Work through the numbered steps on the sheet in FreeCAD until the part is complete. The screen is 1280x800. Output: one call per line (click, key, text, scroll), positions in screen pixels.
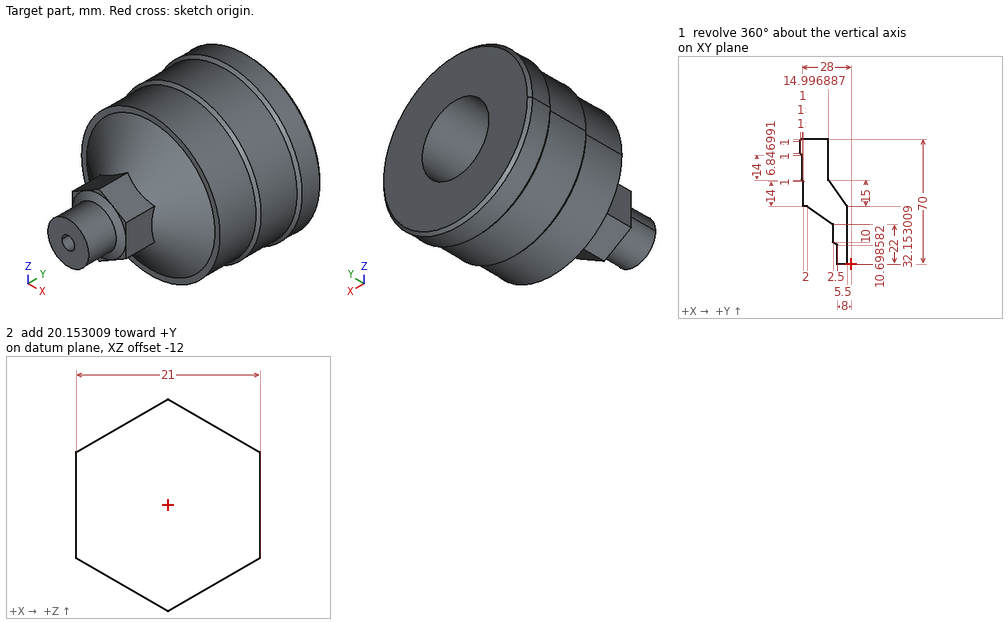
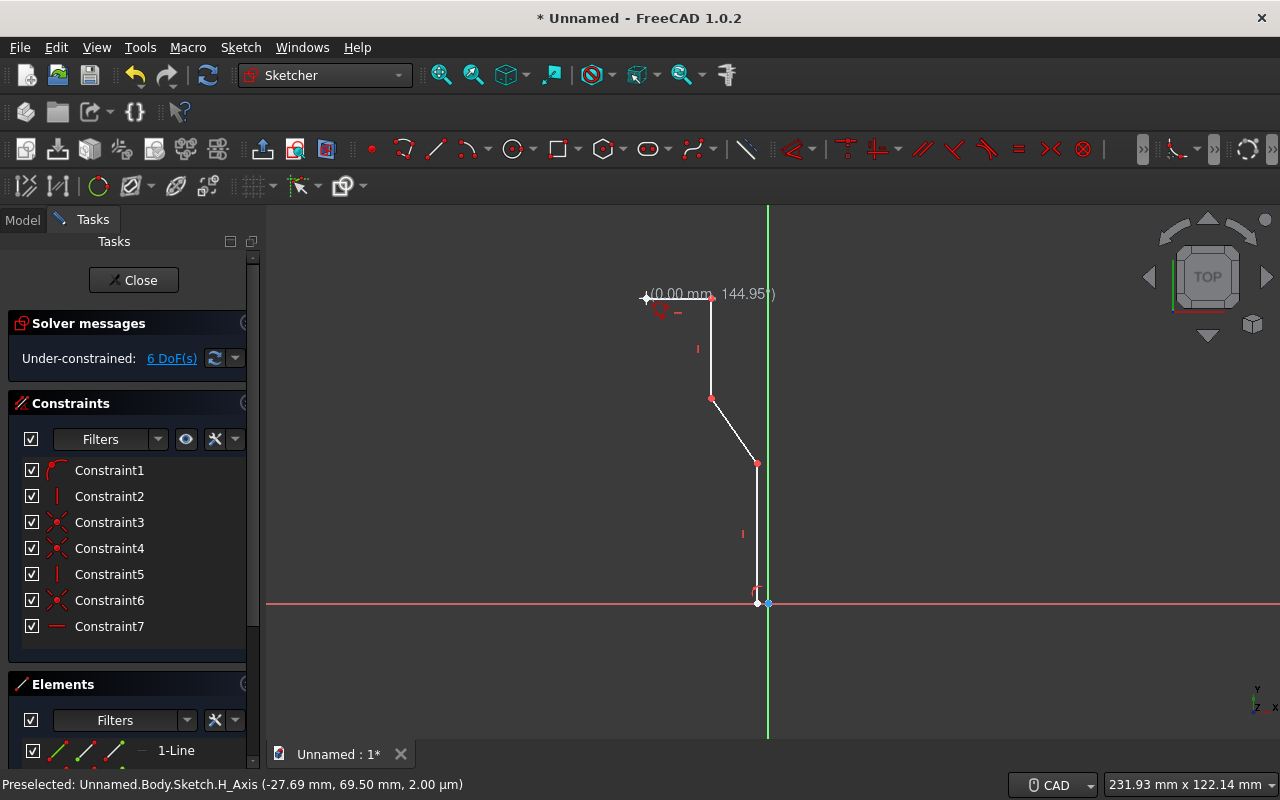
scroll(641, 302, up, 5)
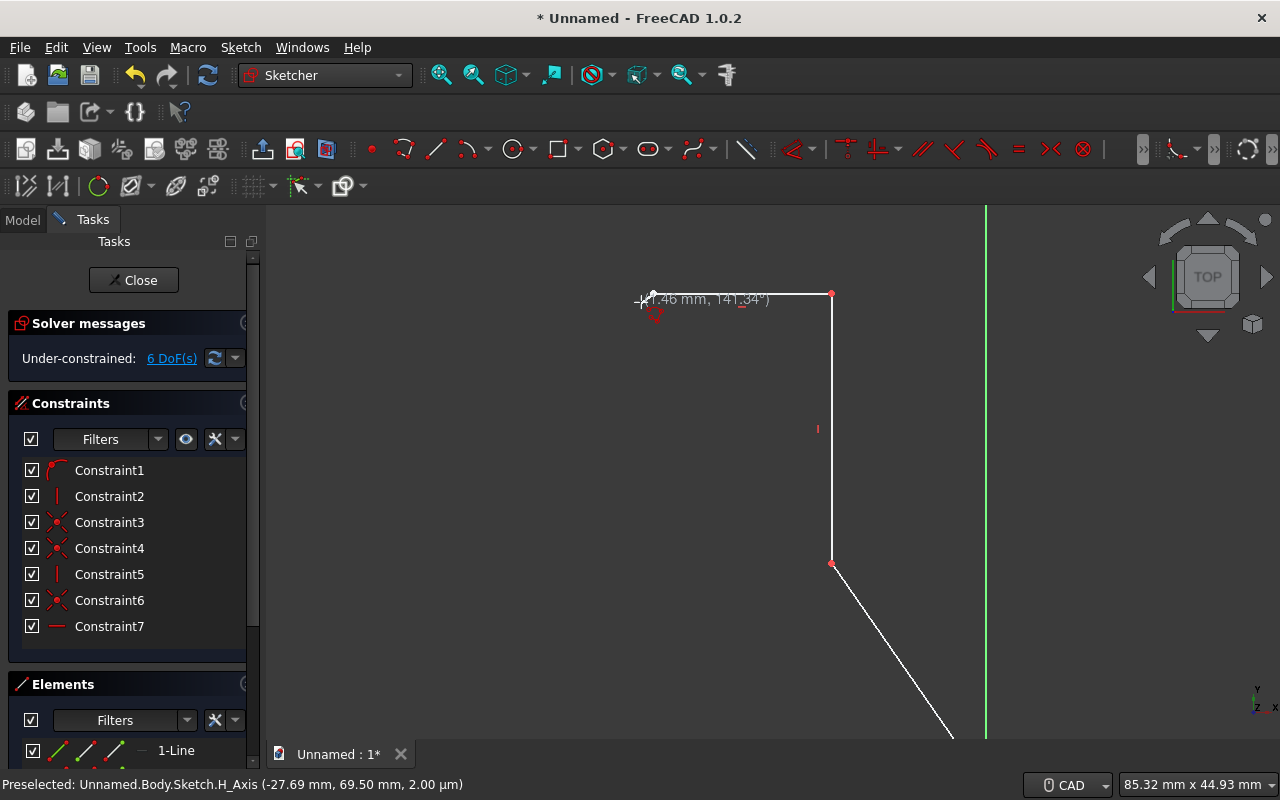
click(641, 302)
click(641, 384)
click(653, 395)
click(653, 562)
click(665, 574)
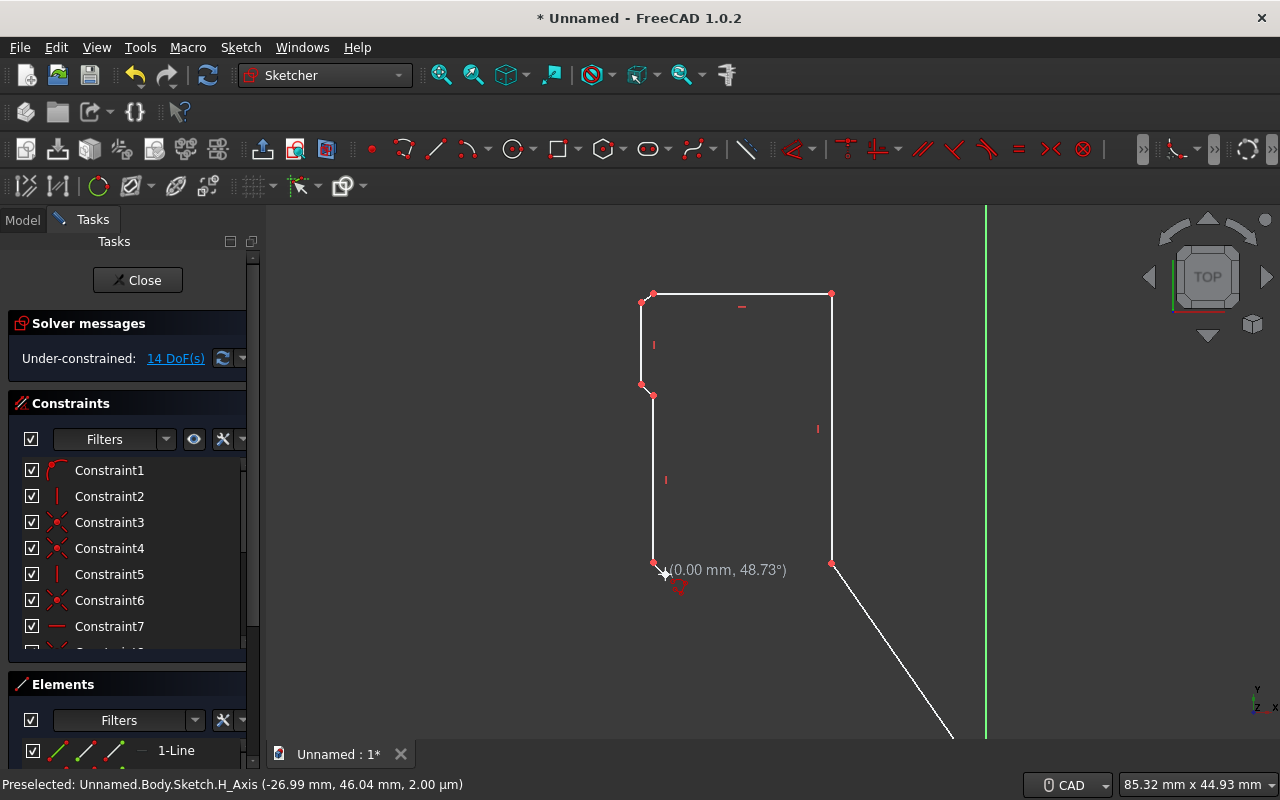
scroll(641, 336, down, 5)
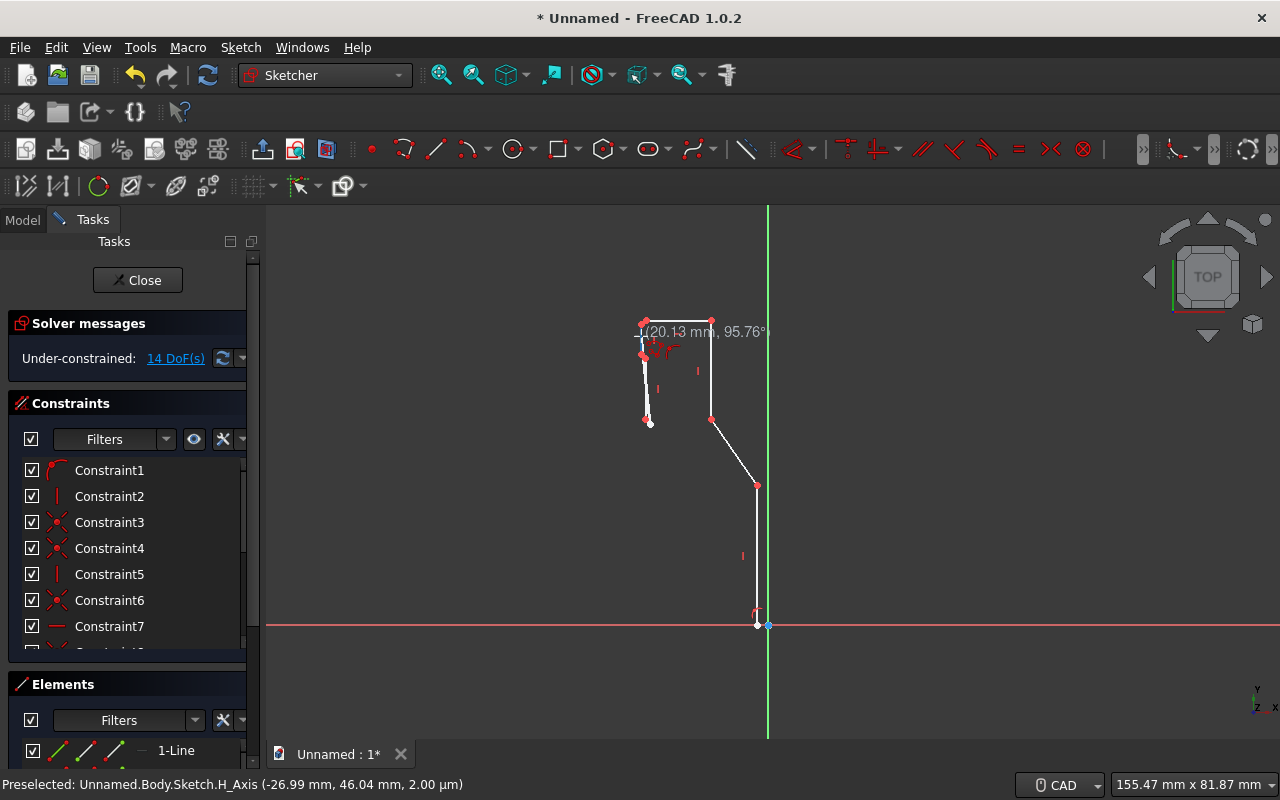
click(650, 485)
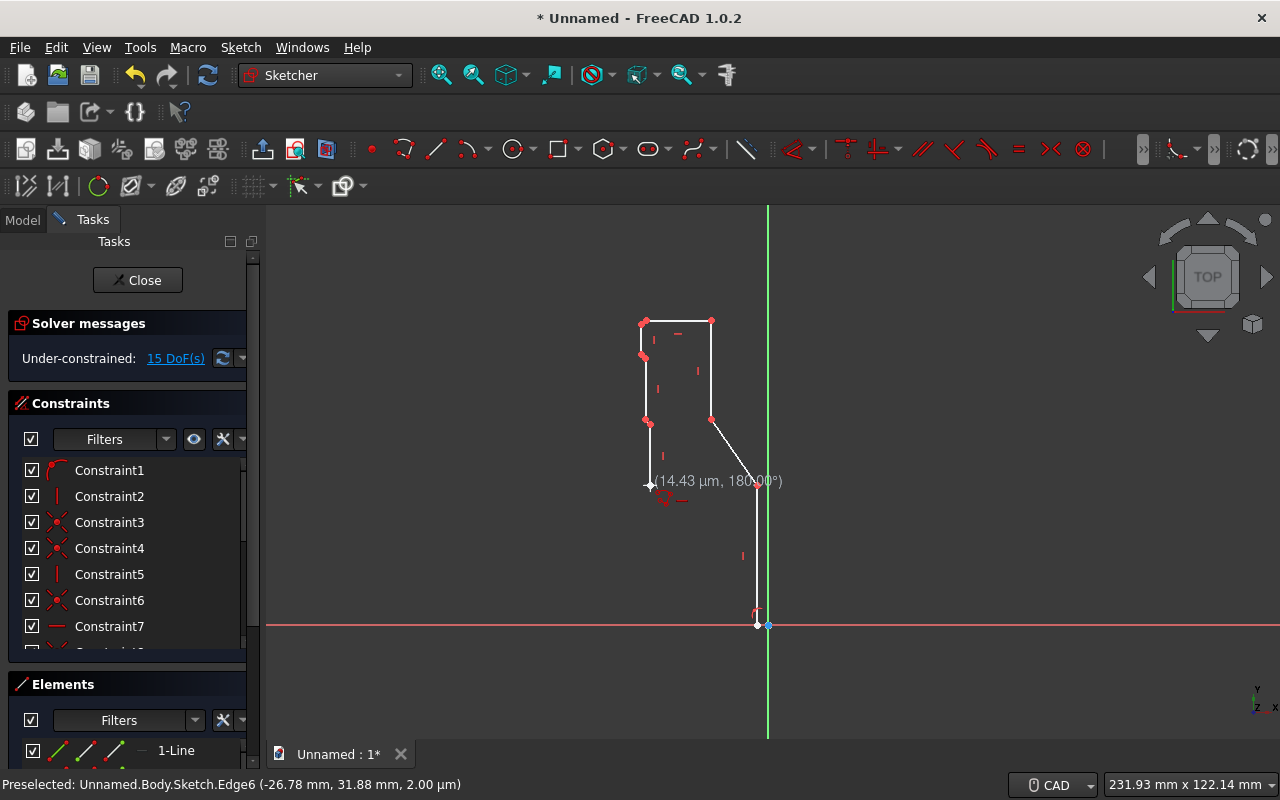
scroll(659, 485, up, 3)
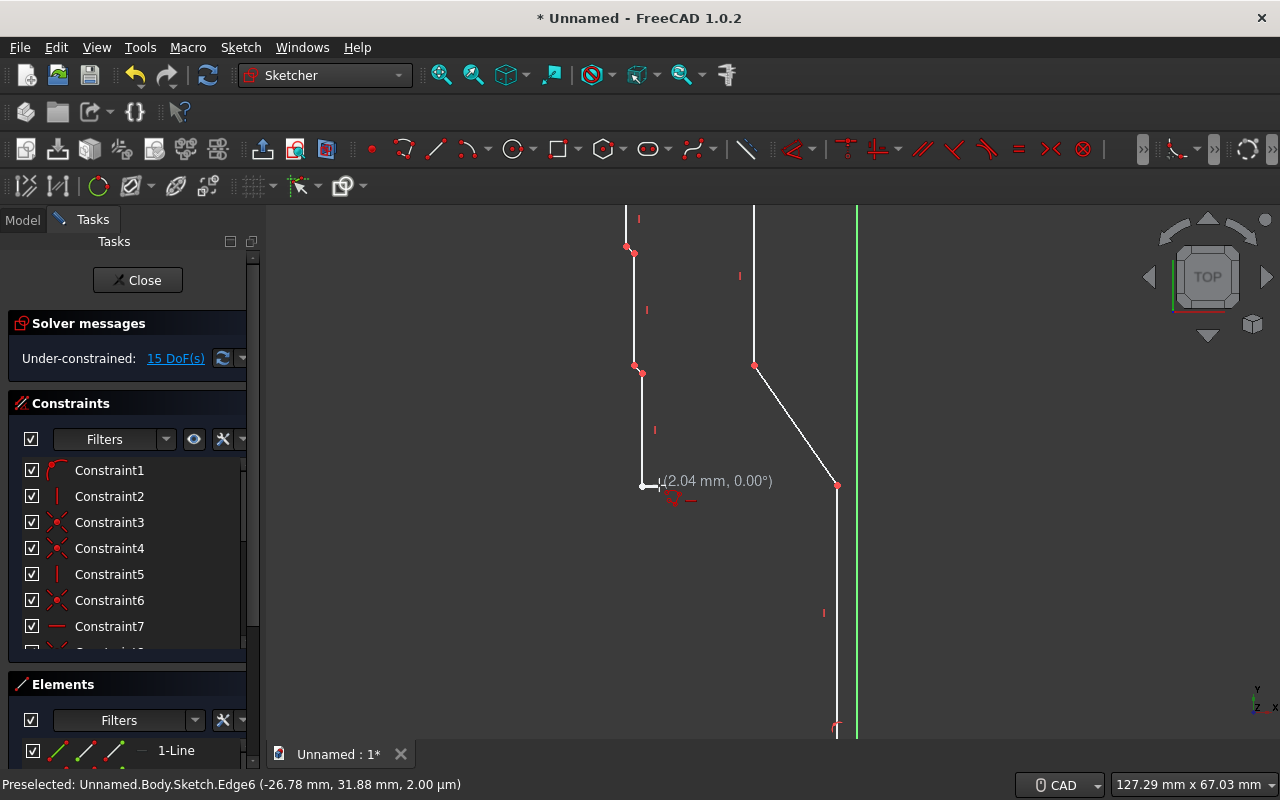
click(658, 485)
click(774, 565)
click(774, 645)
click(794, 655)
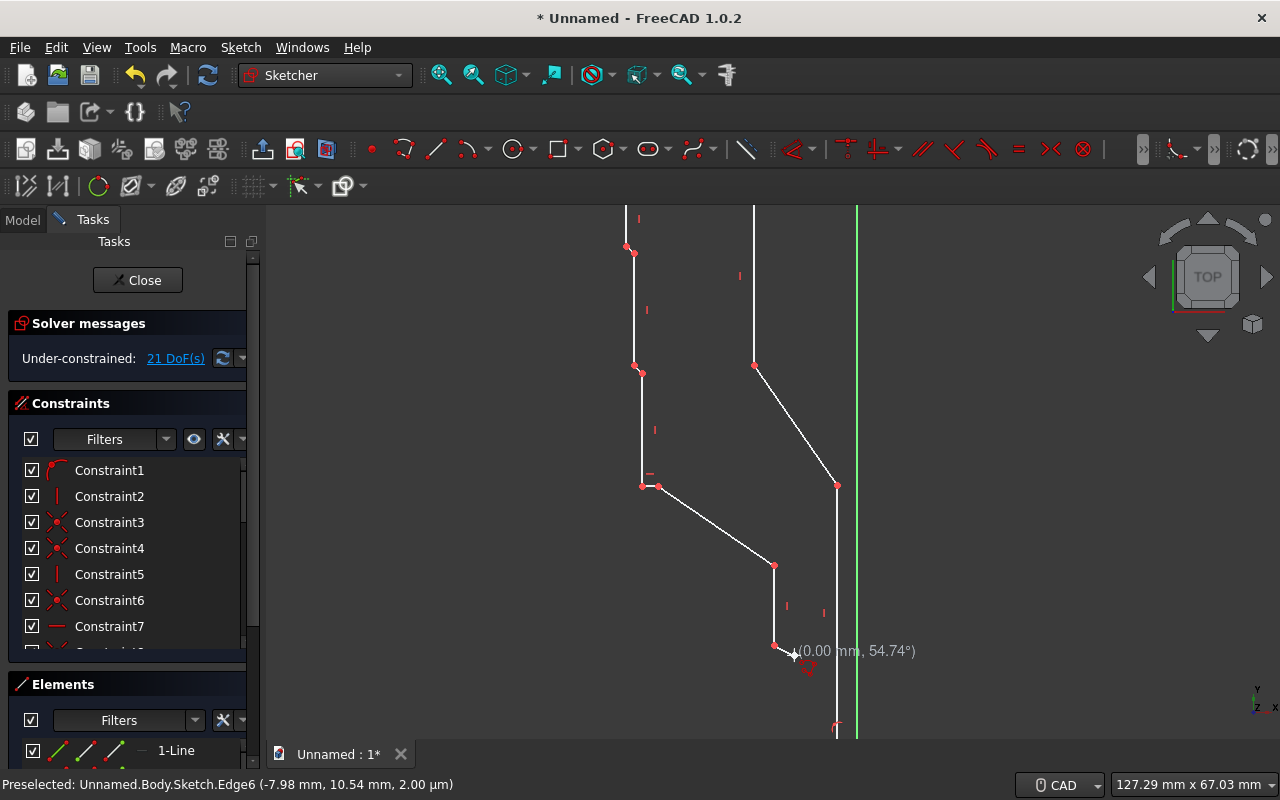
scroll(659, 485, down, 3)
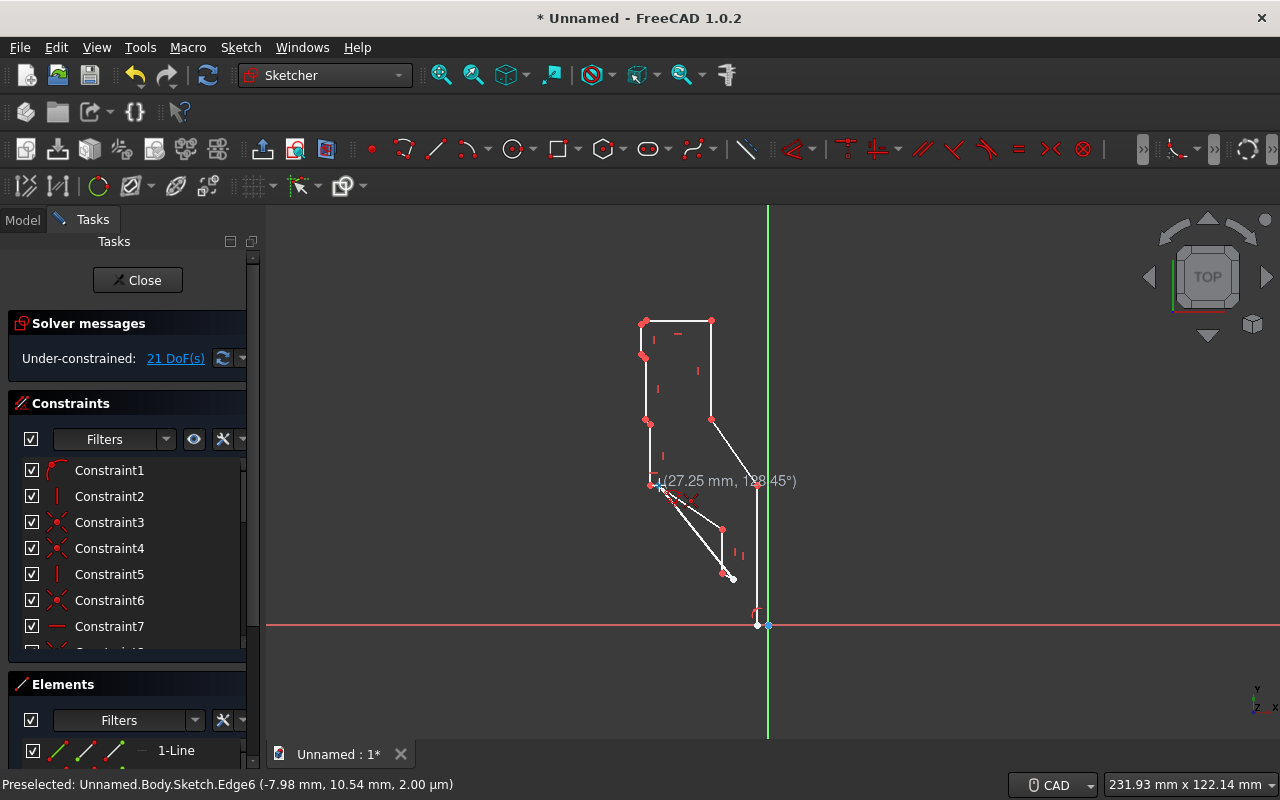
click(733, 616)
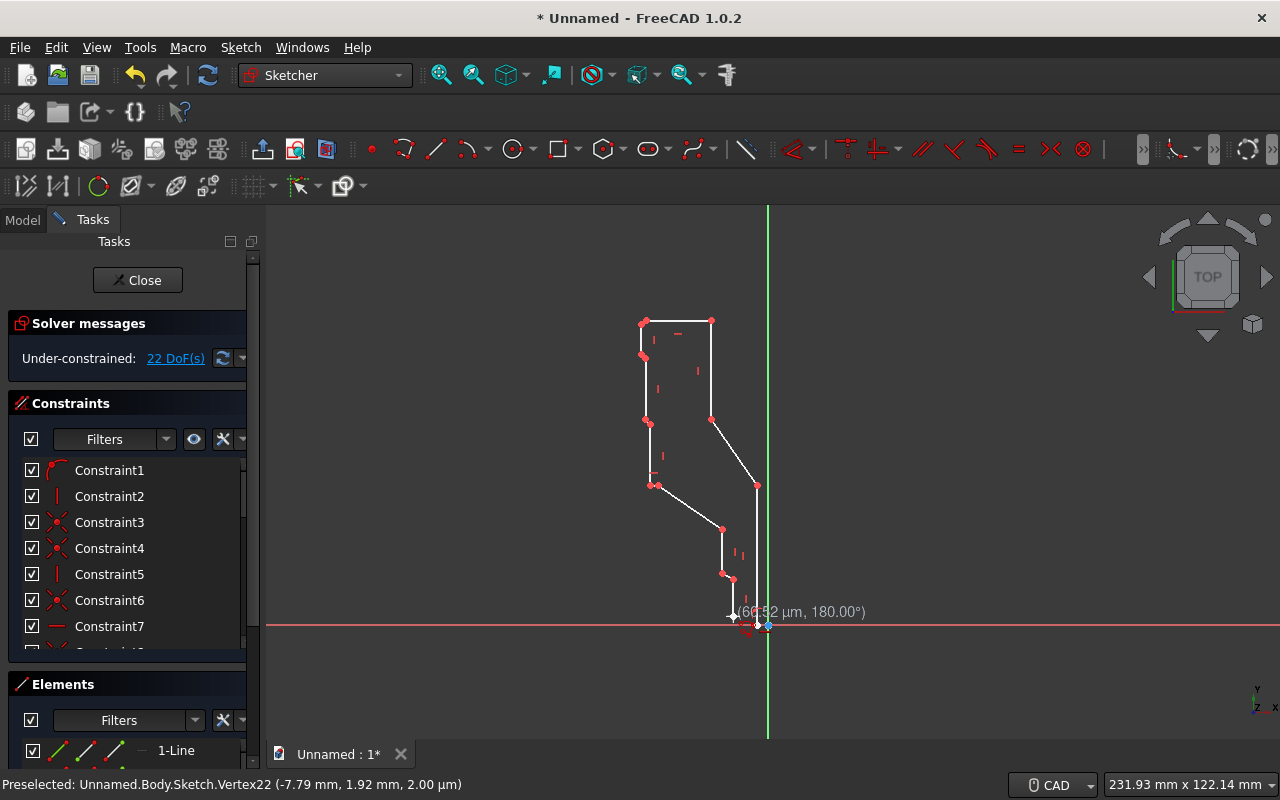
scroll(757, 625, up, 2)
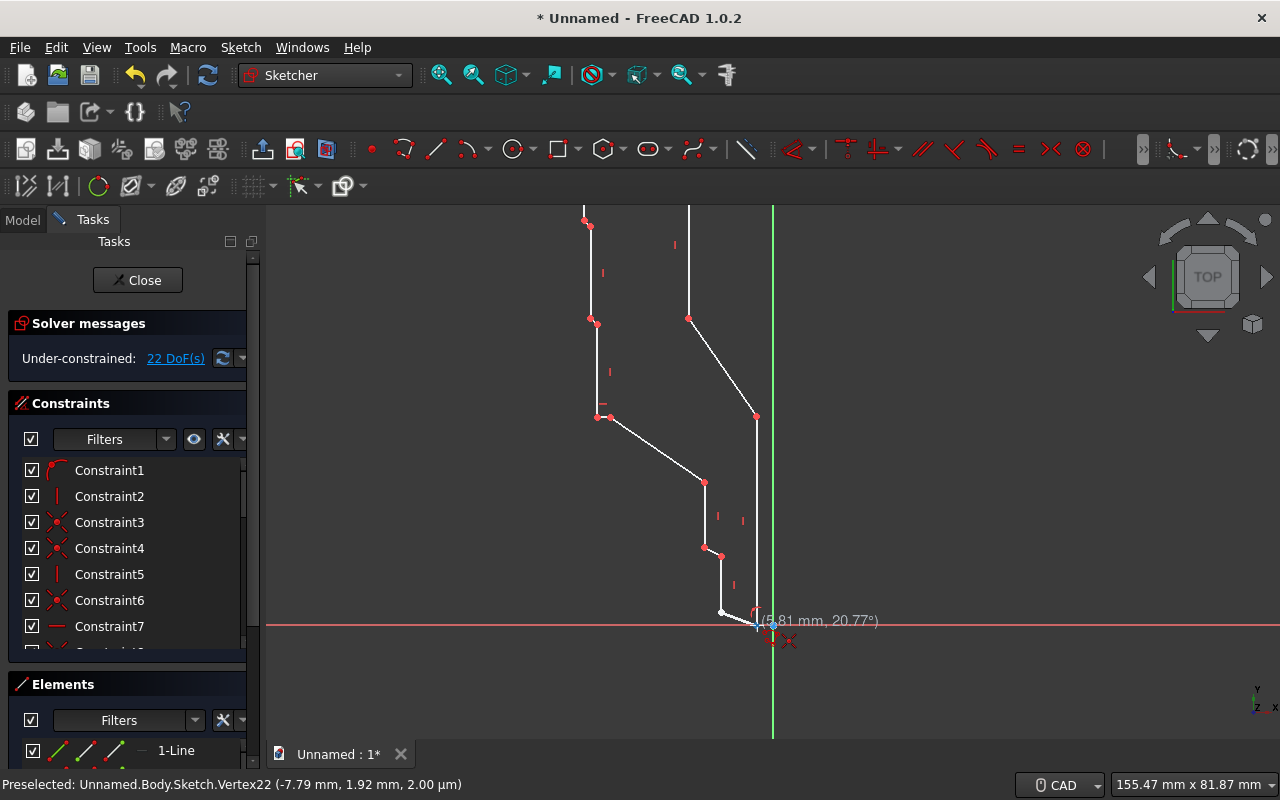
click(757, 625)
key(Escape)
key(Escape)